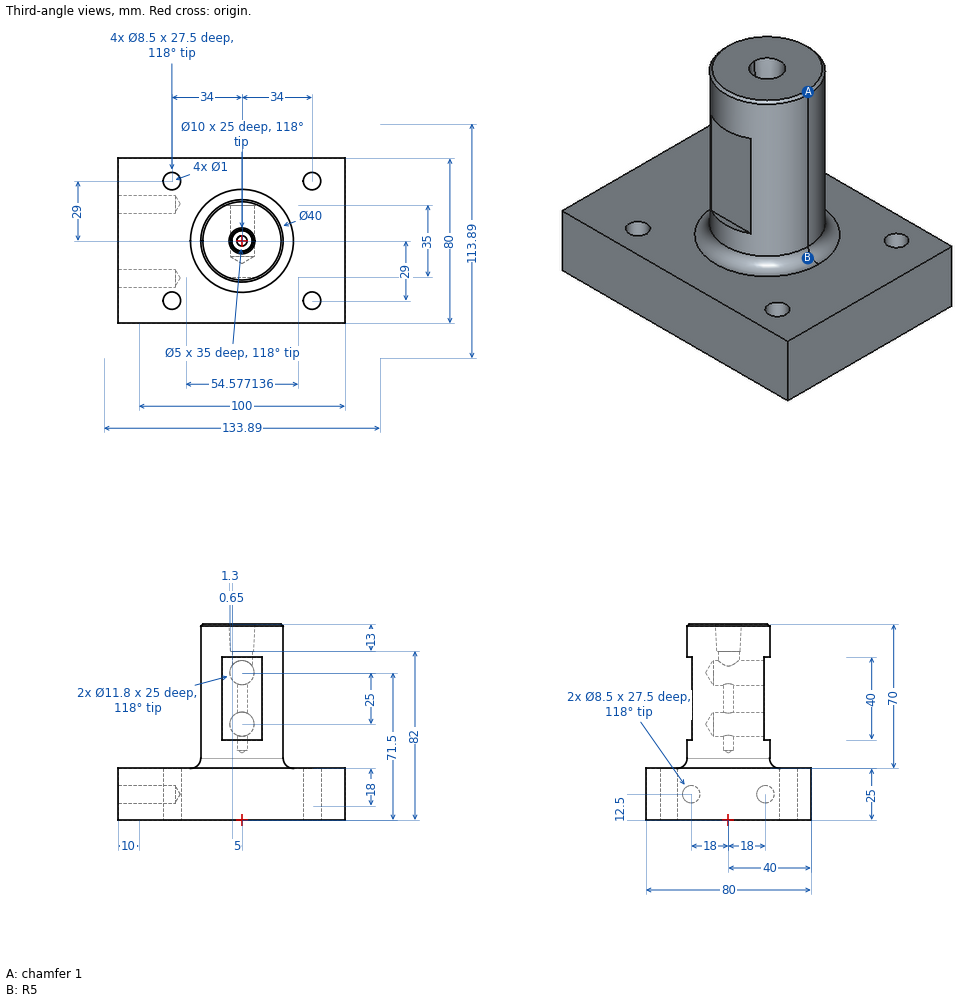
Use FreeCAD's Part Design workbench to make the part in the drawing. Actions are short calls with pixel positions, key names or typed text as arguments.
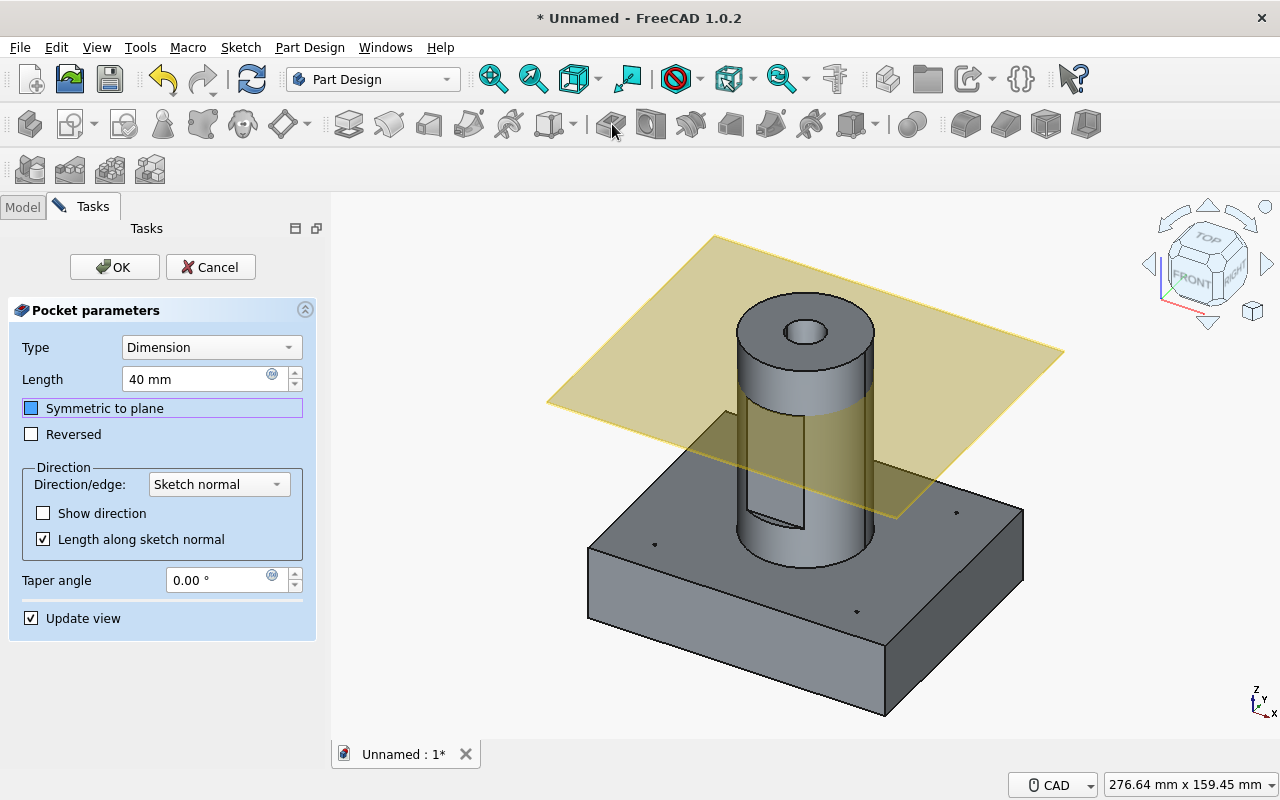
click(115, 267)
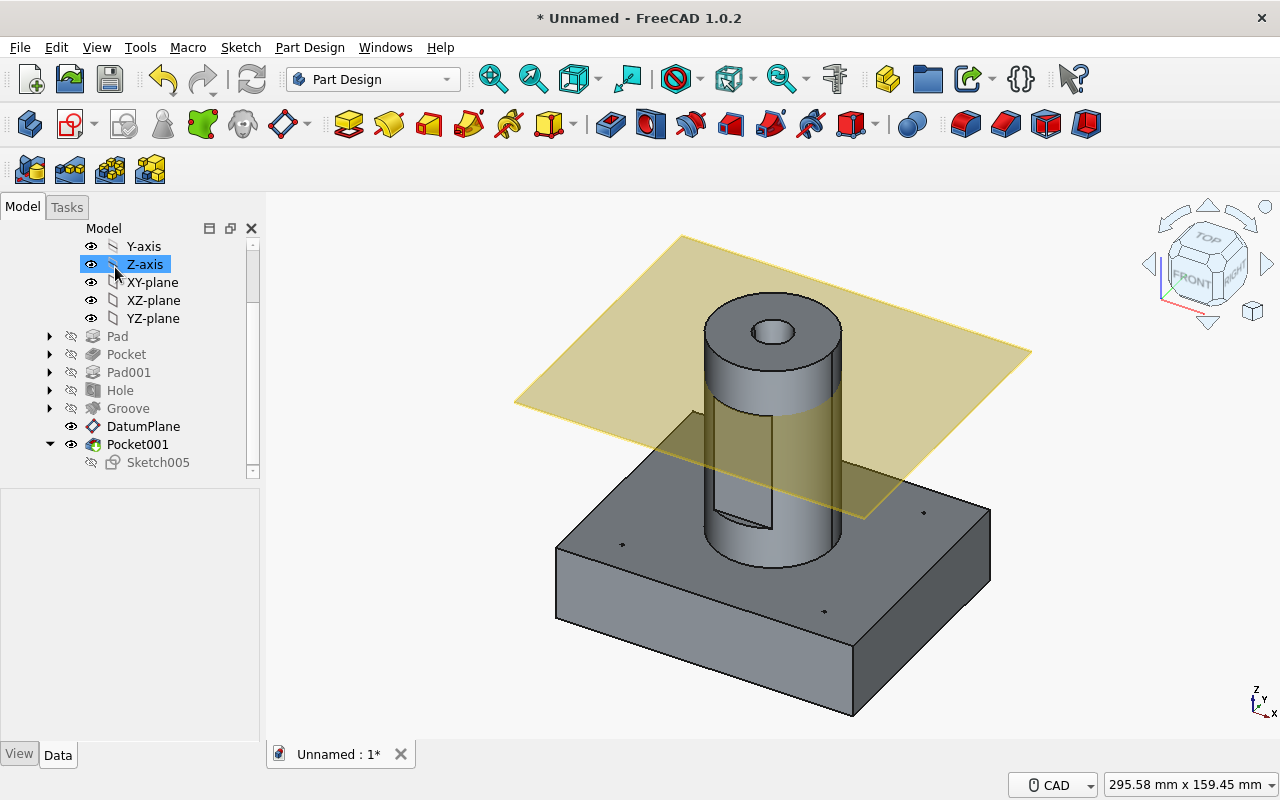
click(116, 426)
key(space)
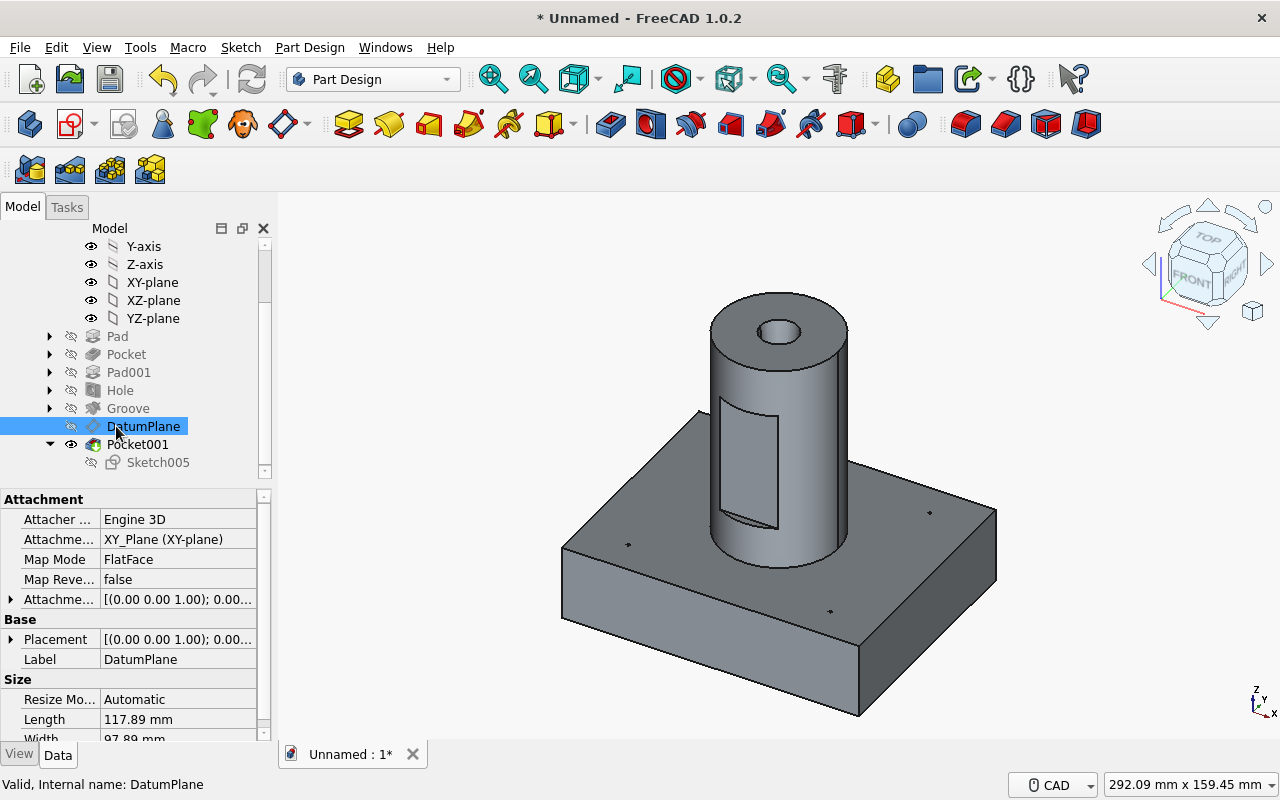
key(4)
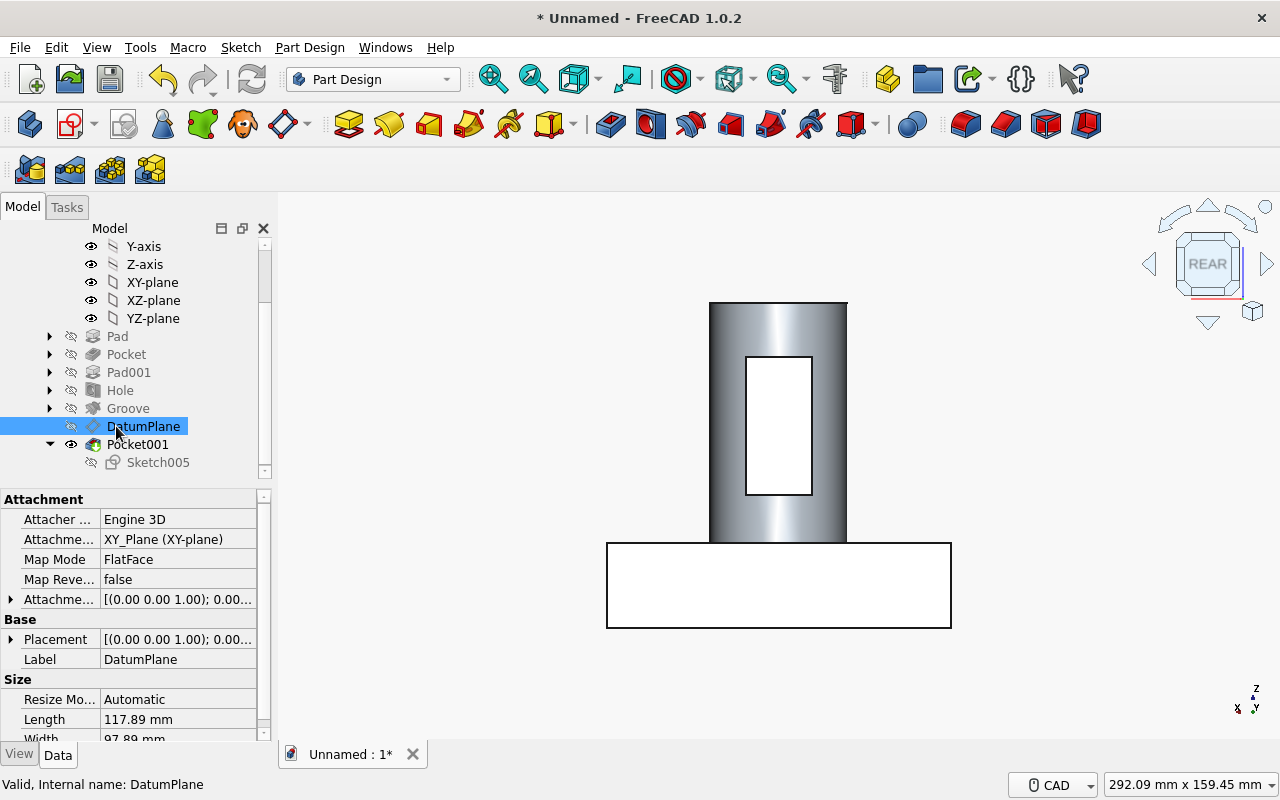
click(779, 405)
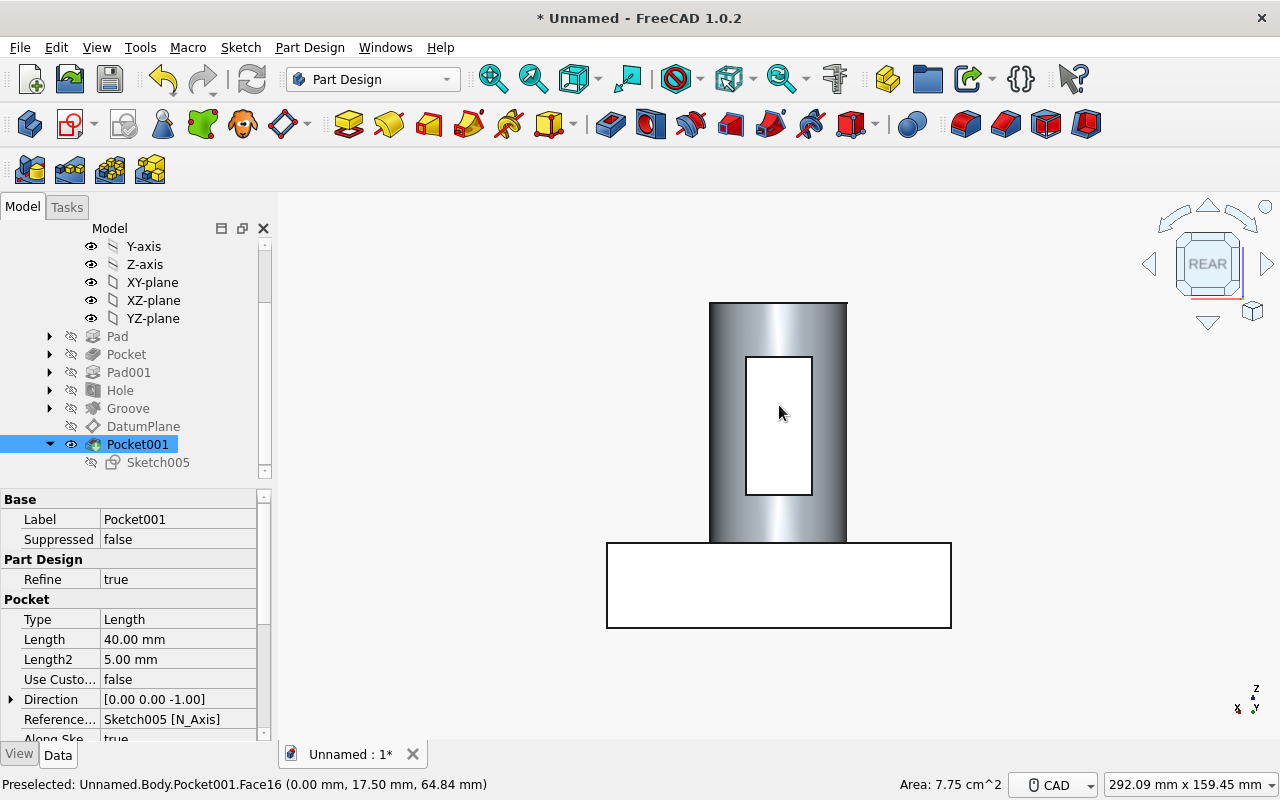
click(70, 124)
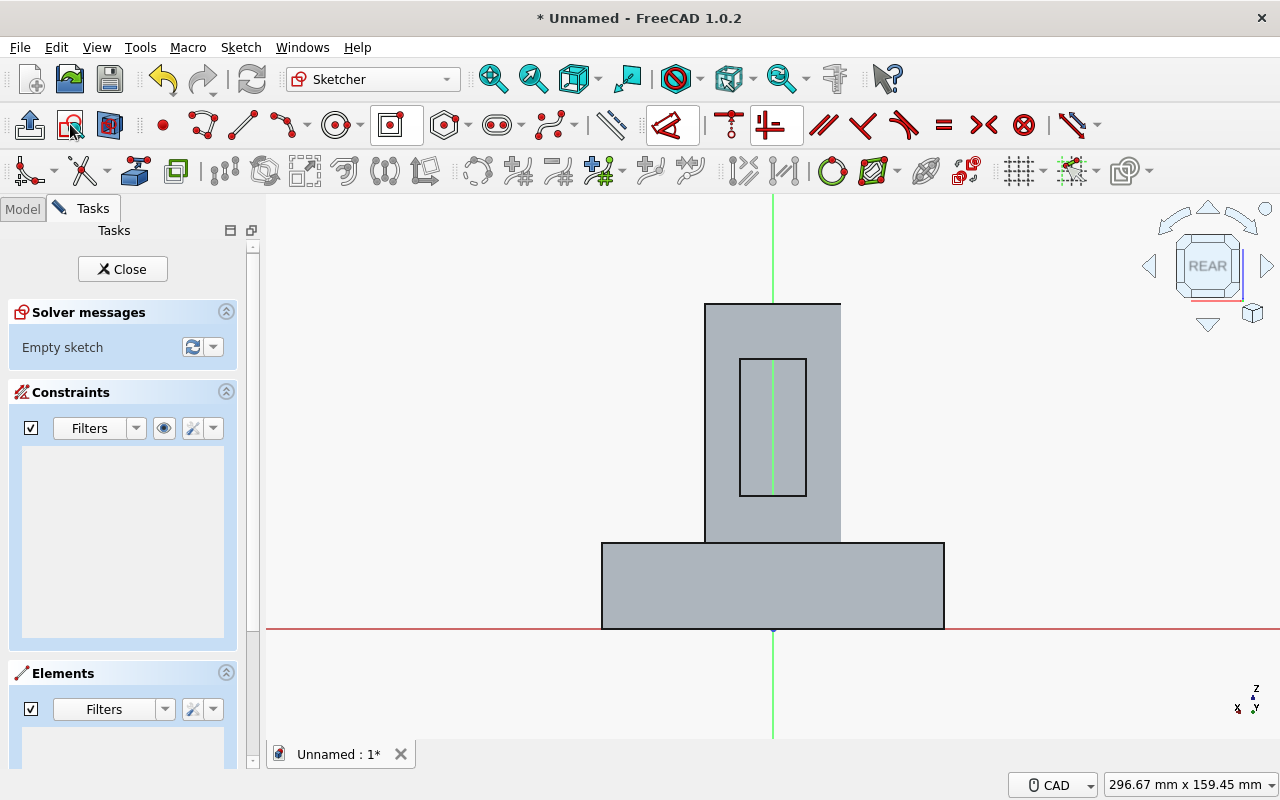
click(336, 126)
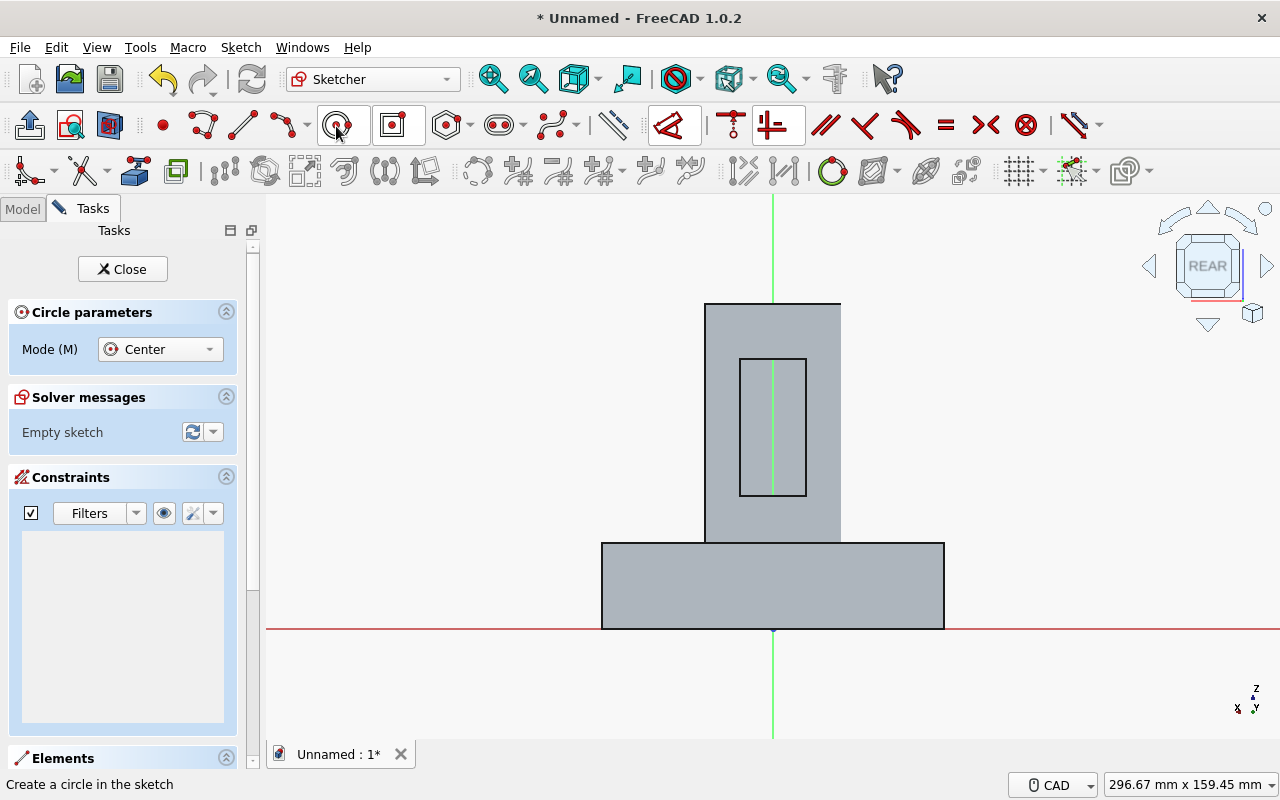
click(773, 384)
click(787, 370)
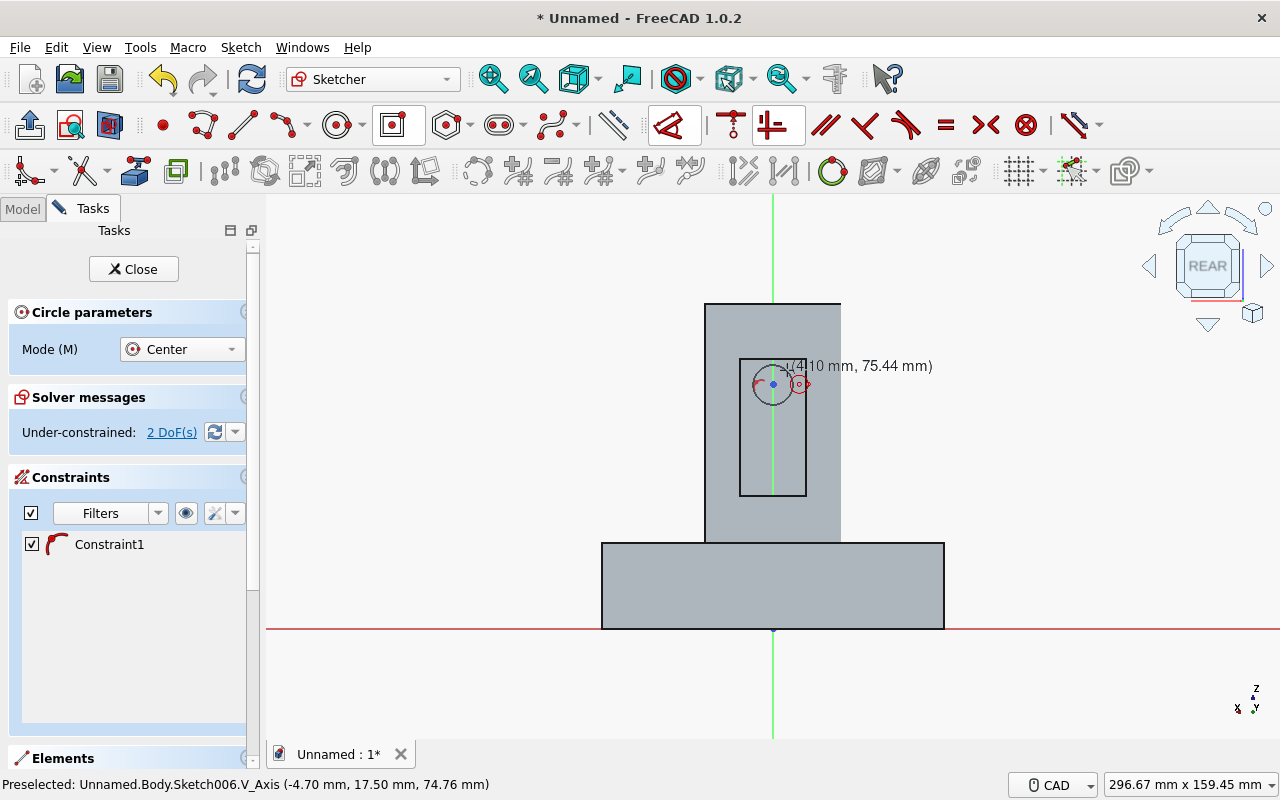
click(773, 470)
click(787, 456)
key(Escape)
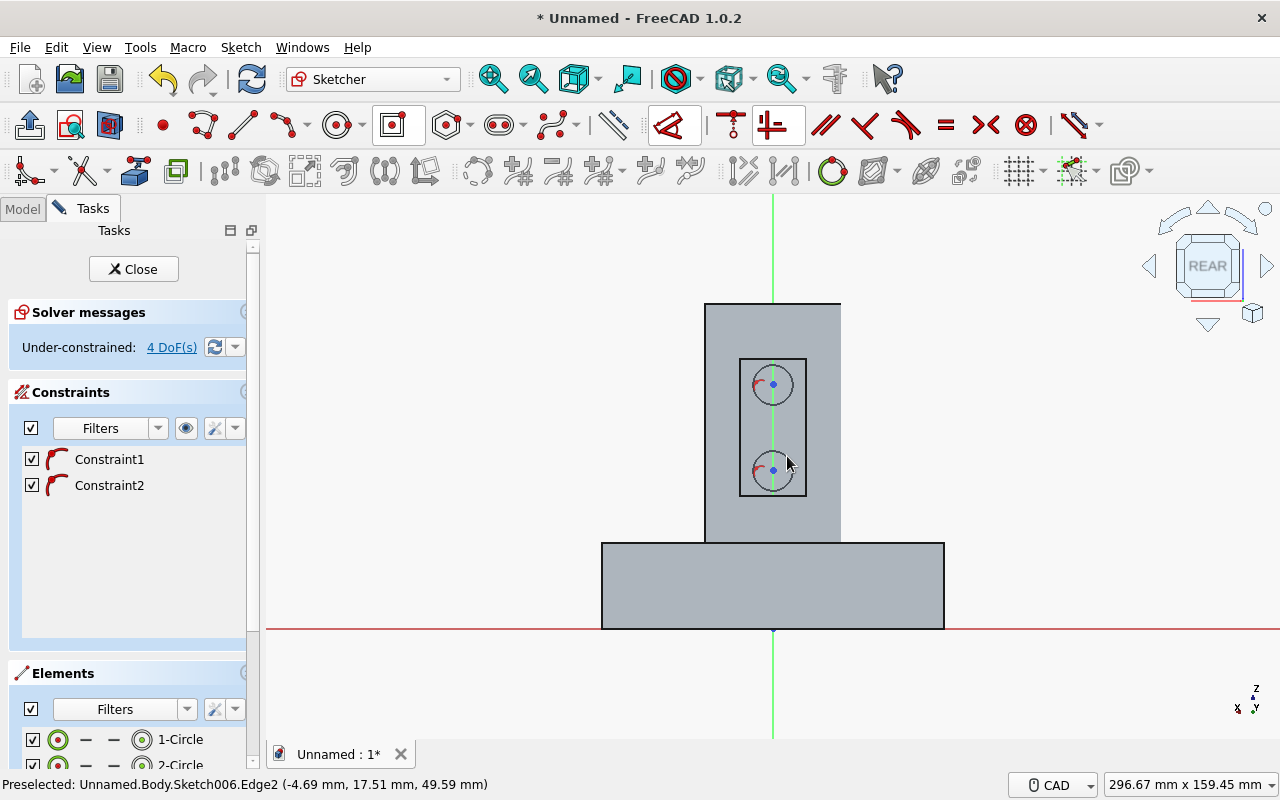
click(787, 371)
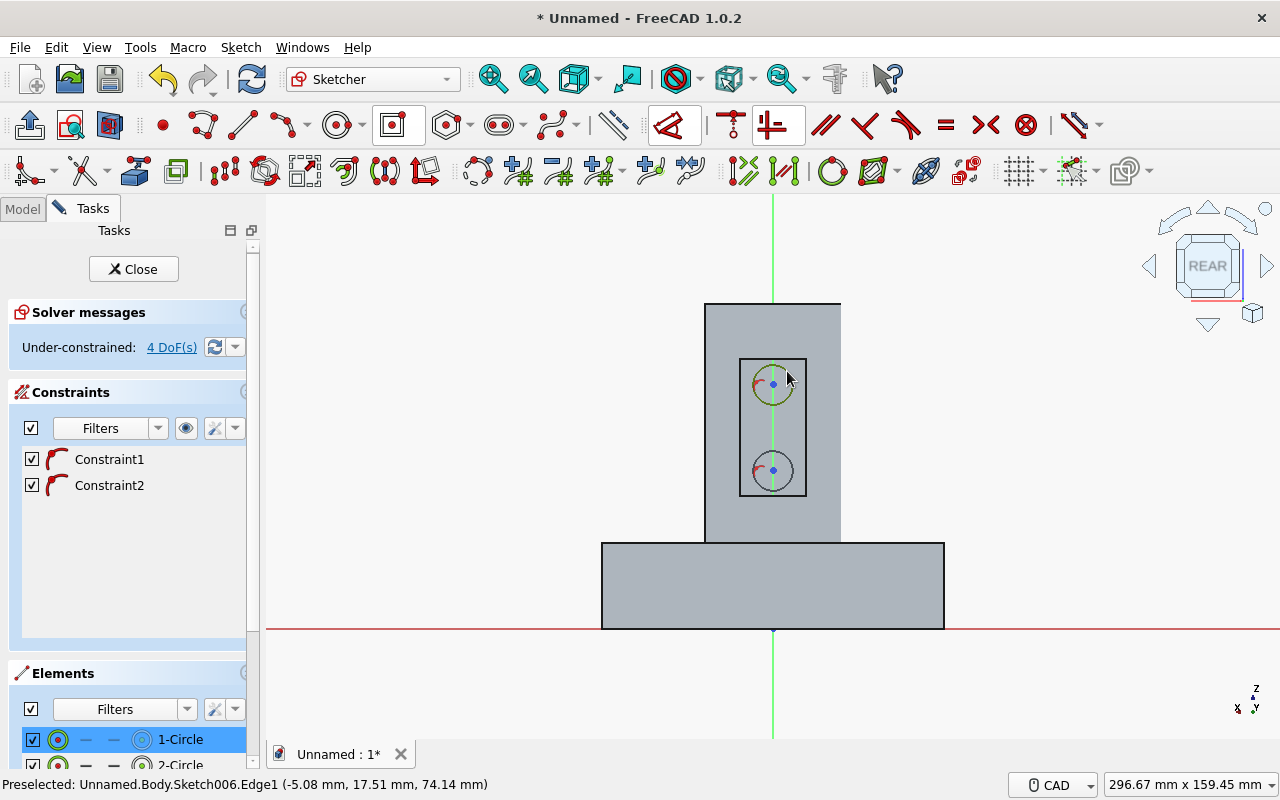
click(787, 457)